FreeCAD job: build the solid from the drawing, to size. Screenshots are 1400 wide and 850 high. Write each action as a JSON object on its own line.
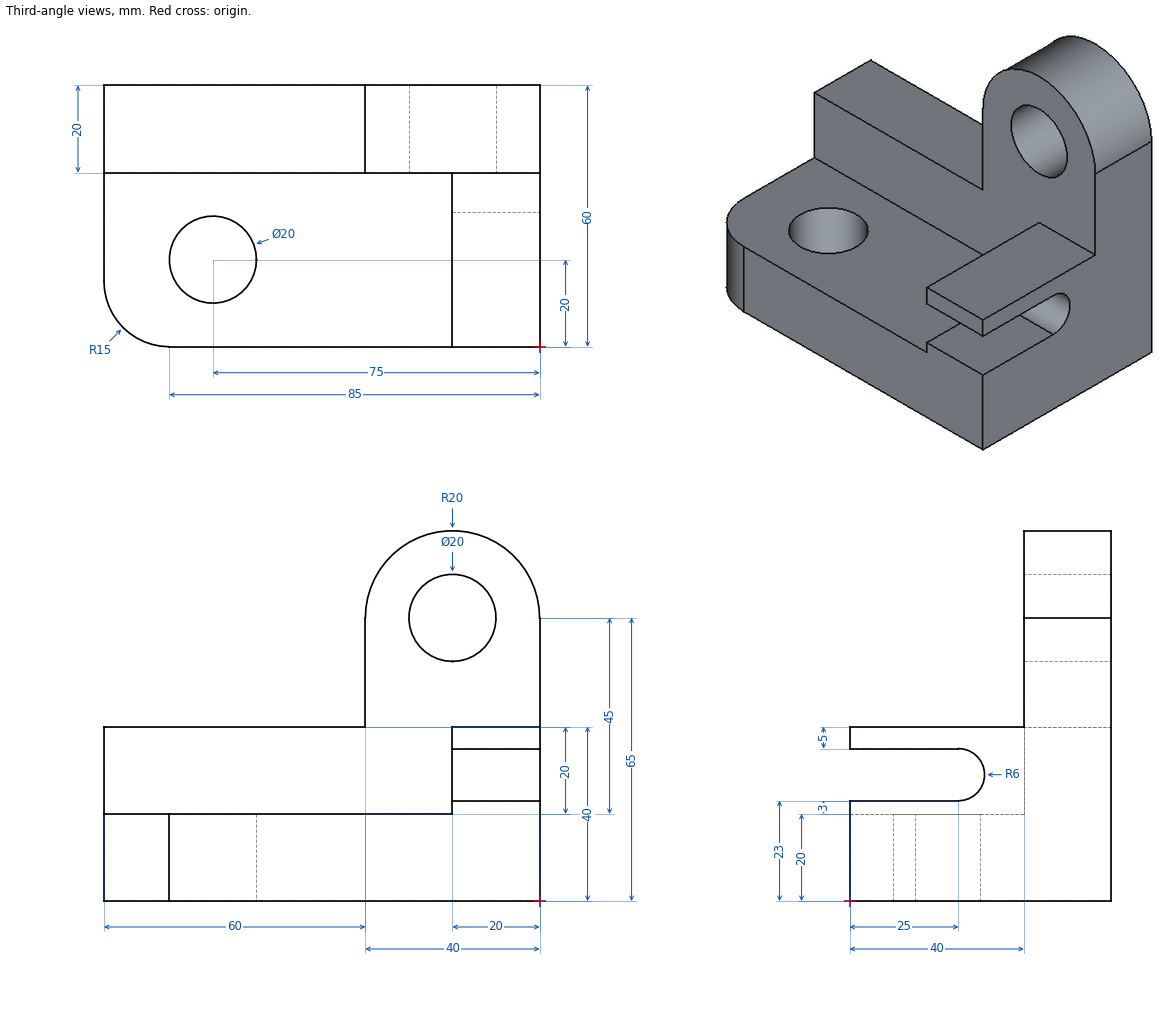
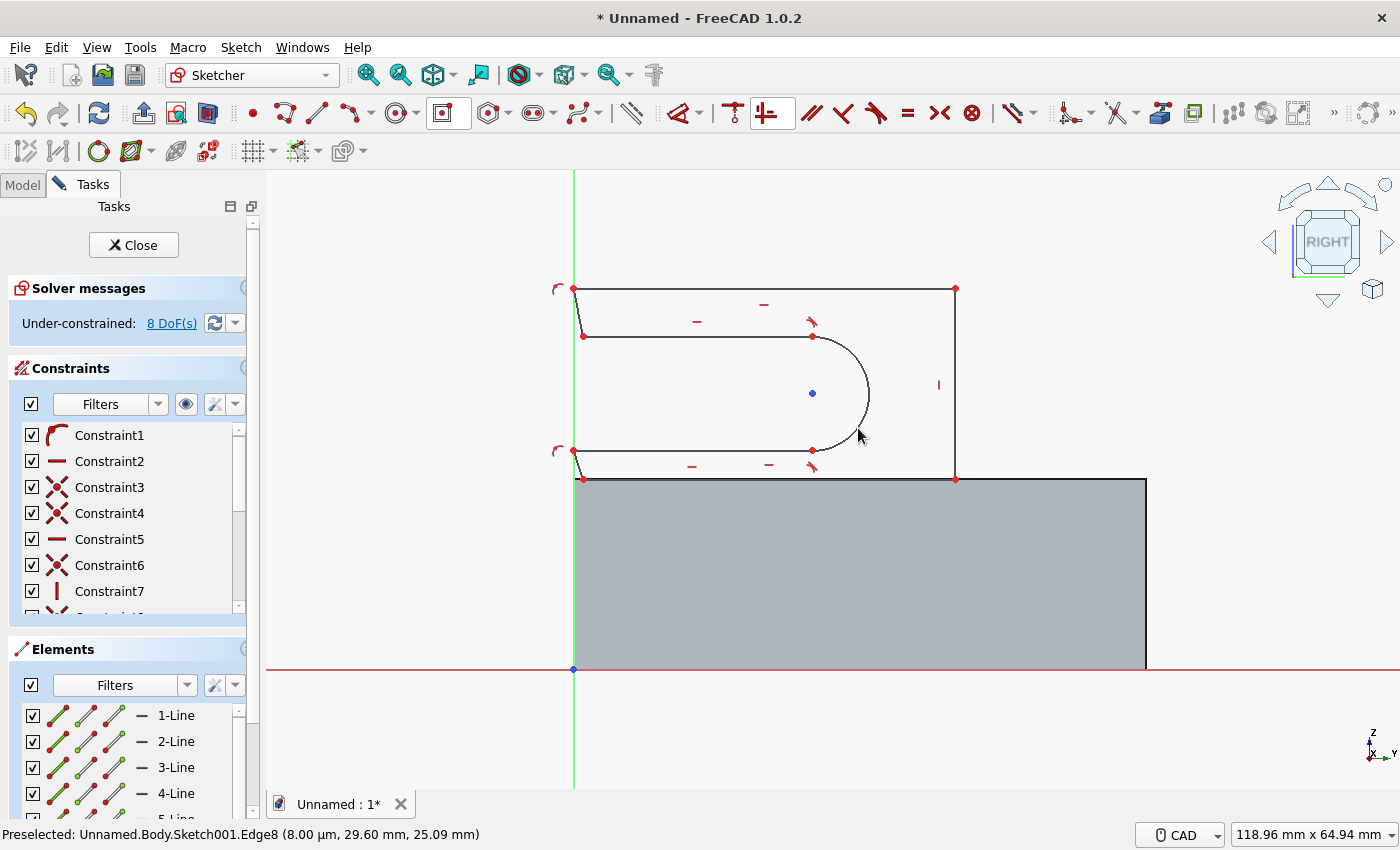
{"action": "left_click", "coordinate": [577, 463]}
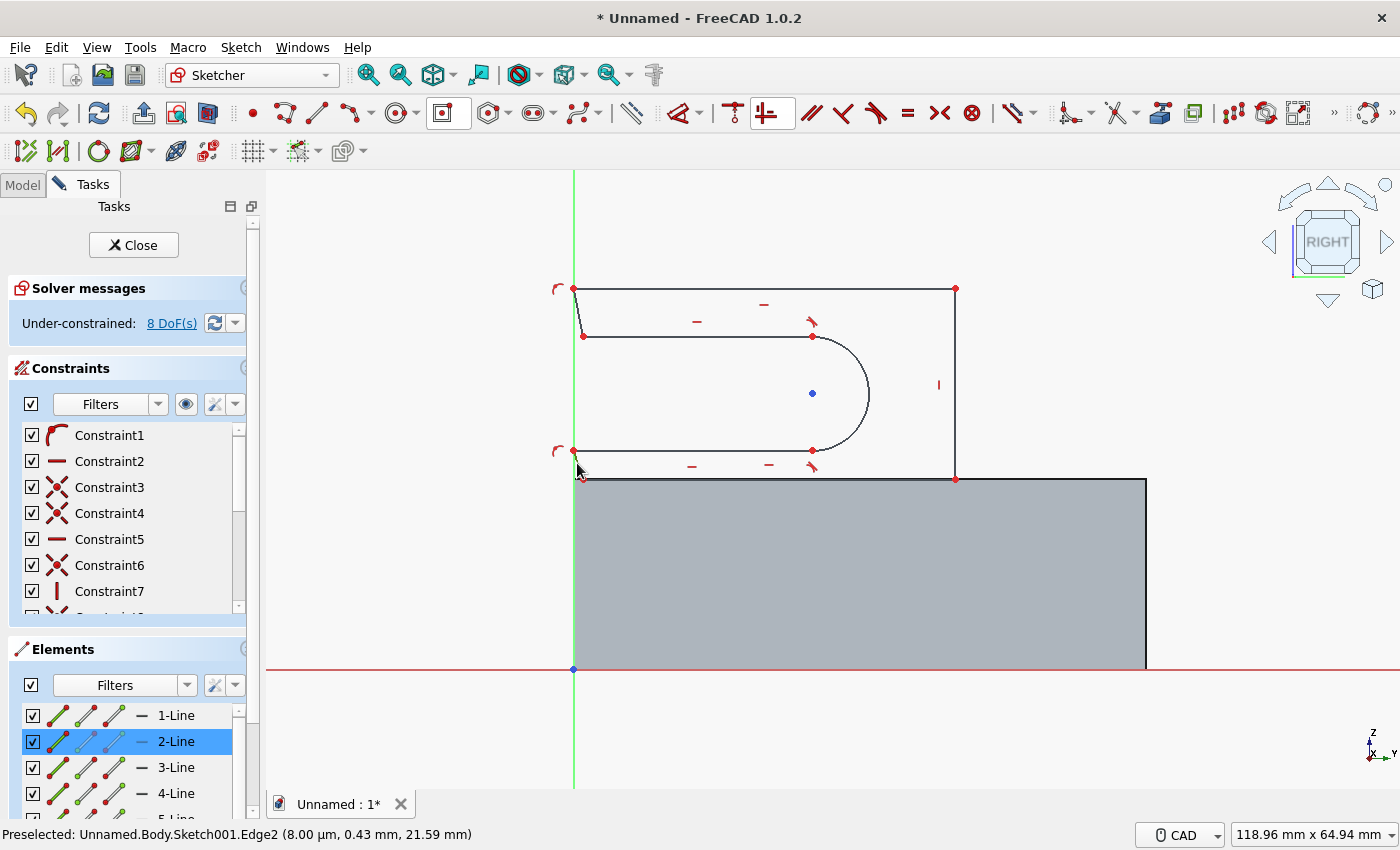
{"action": "key", "text": "v"}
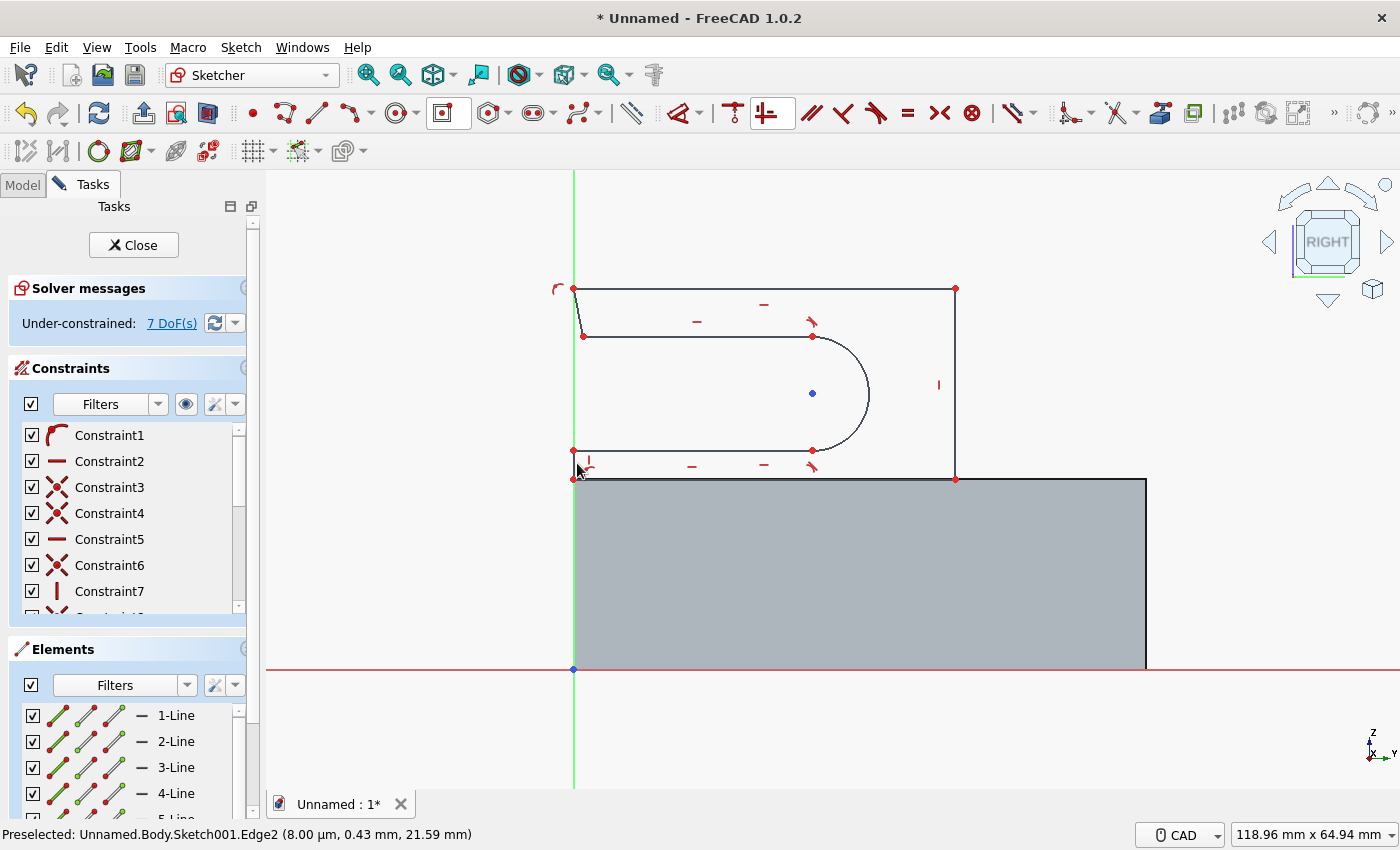
{"action": "left_click", "coordinate": [577, 303]}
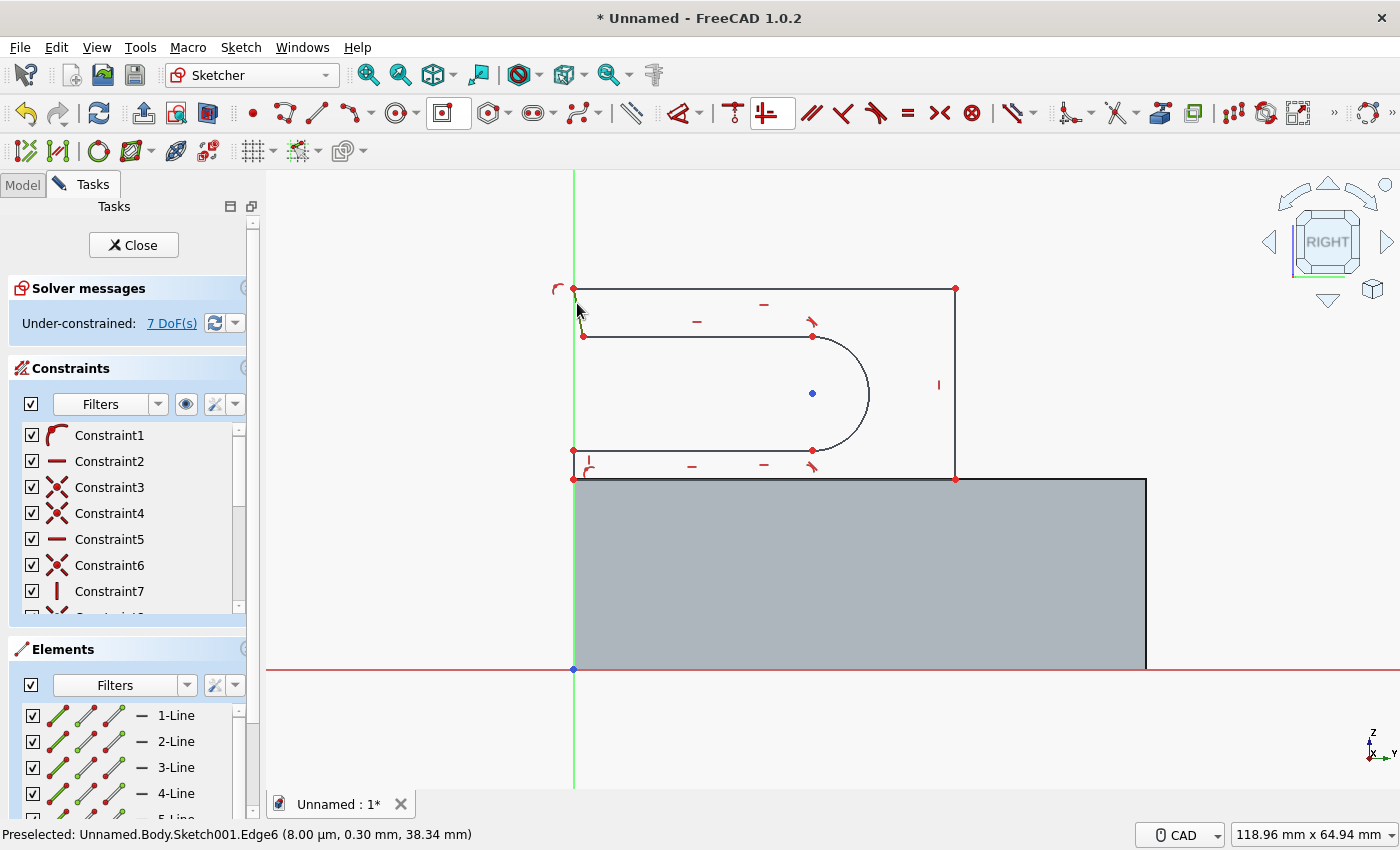
{"action": "key", "text": "v"}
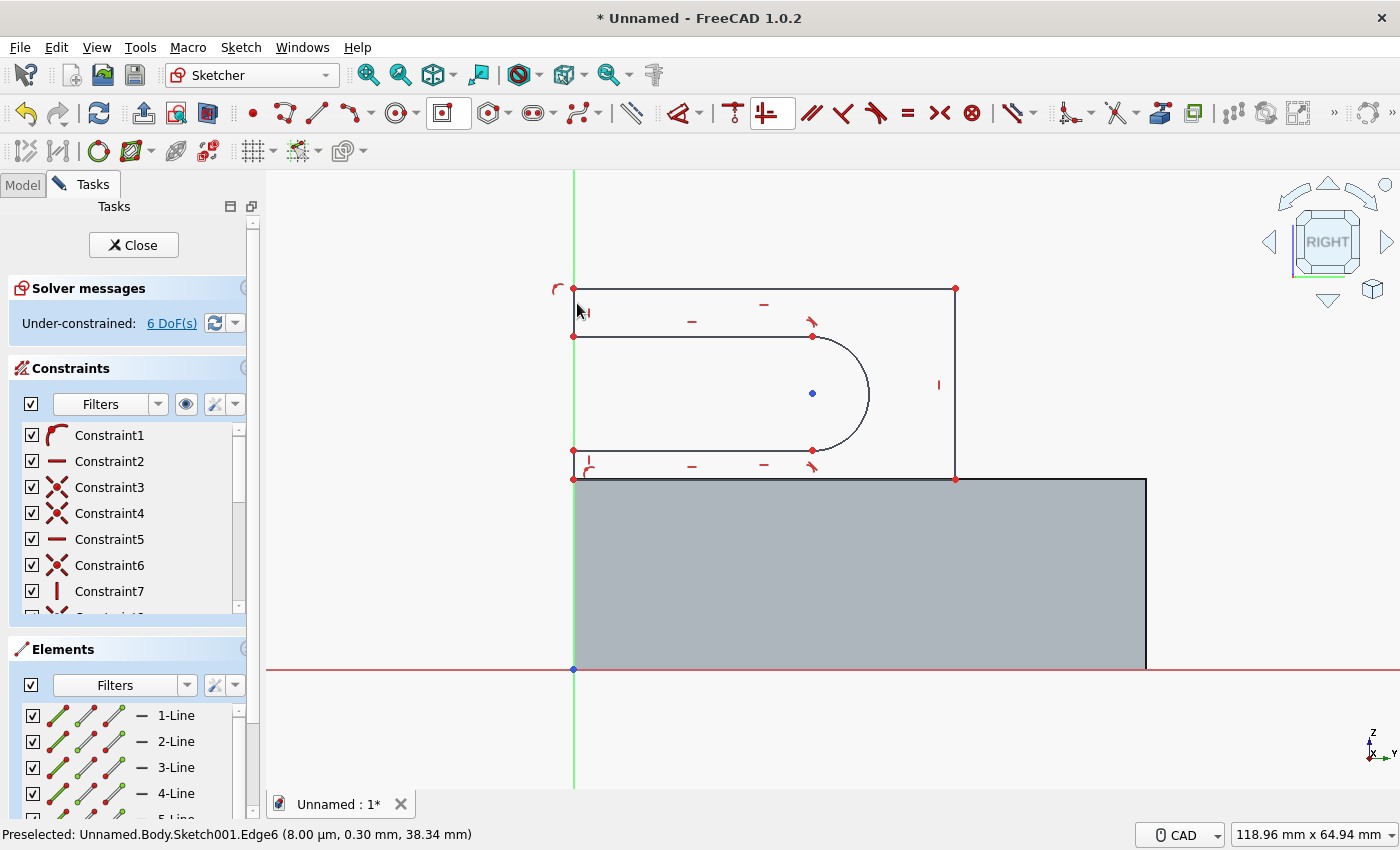
{"action": "key", "text": "d"}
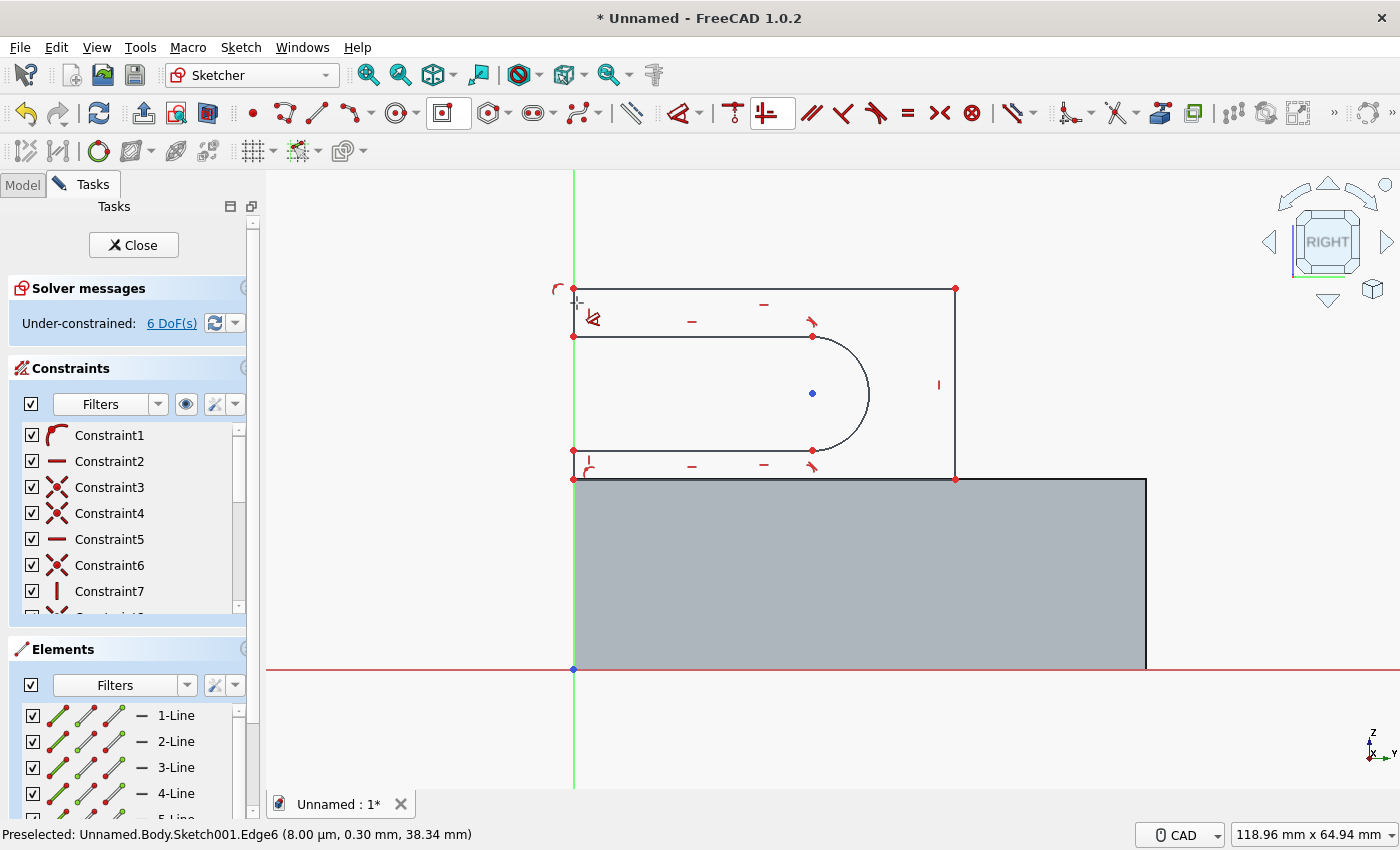
{"action": "left_click", "coordinate": [858, 428]}
{"action": "left_click", "coordinate": [884, 447]}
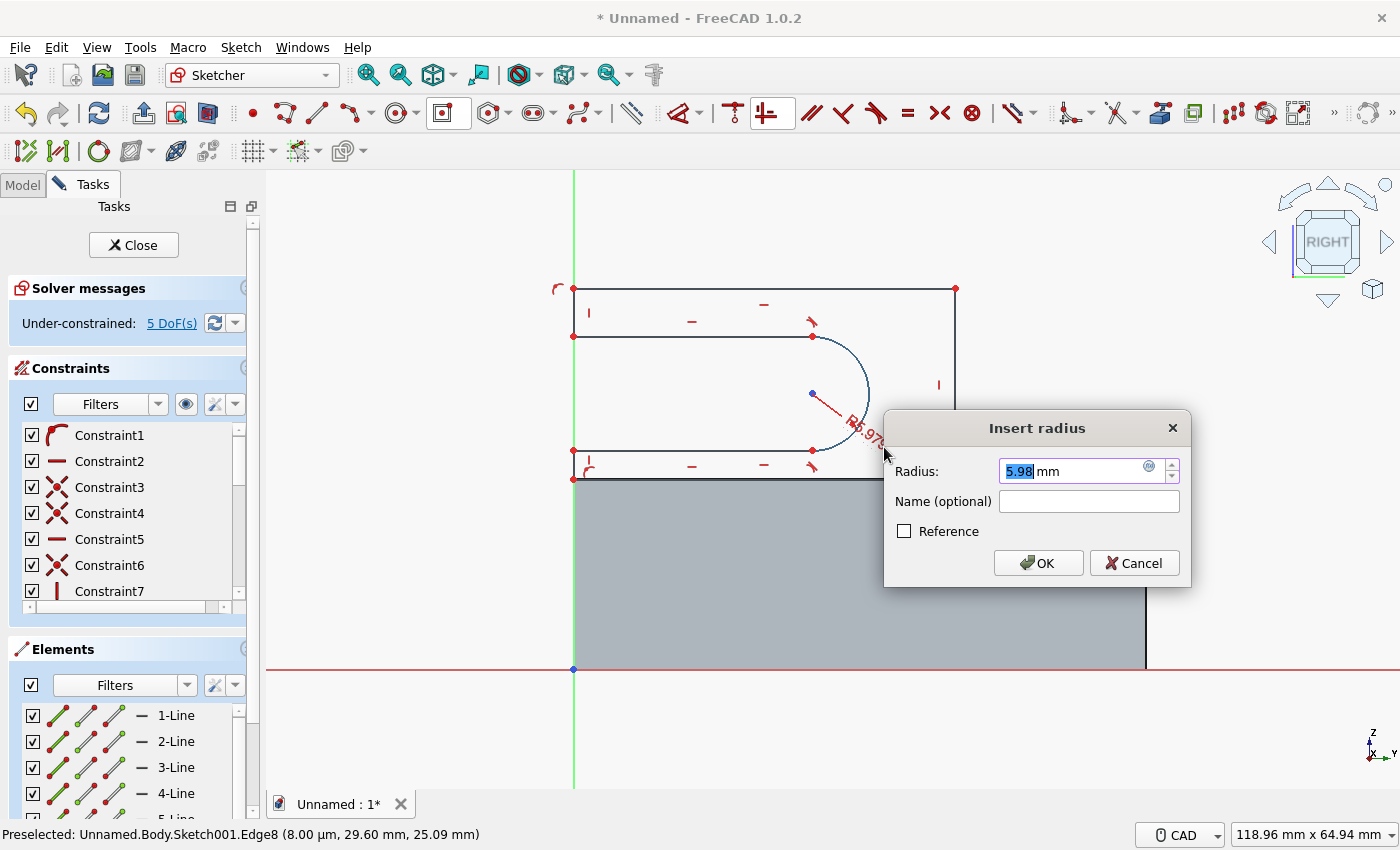
{"action": "type", "text": "6"}
{"action": "key", "text": "Return"}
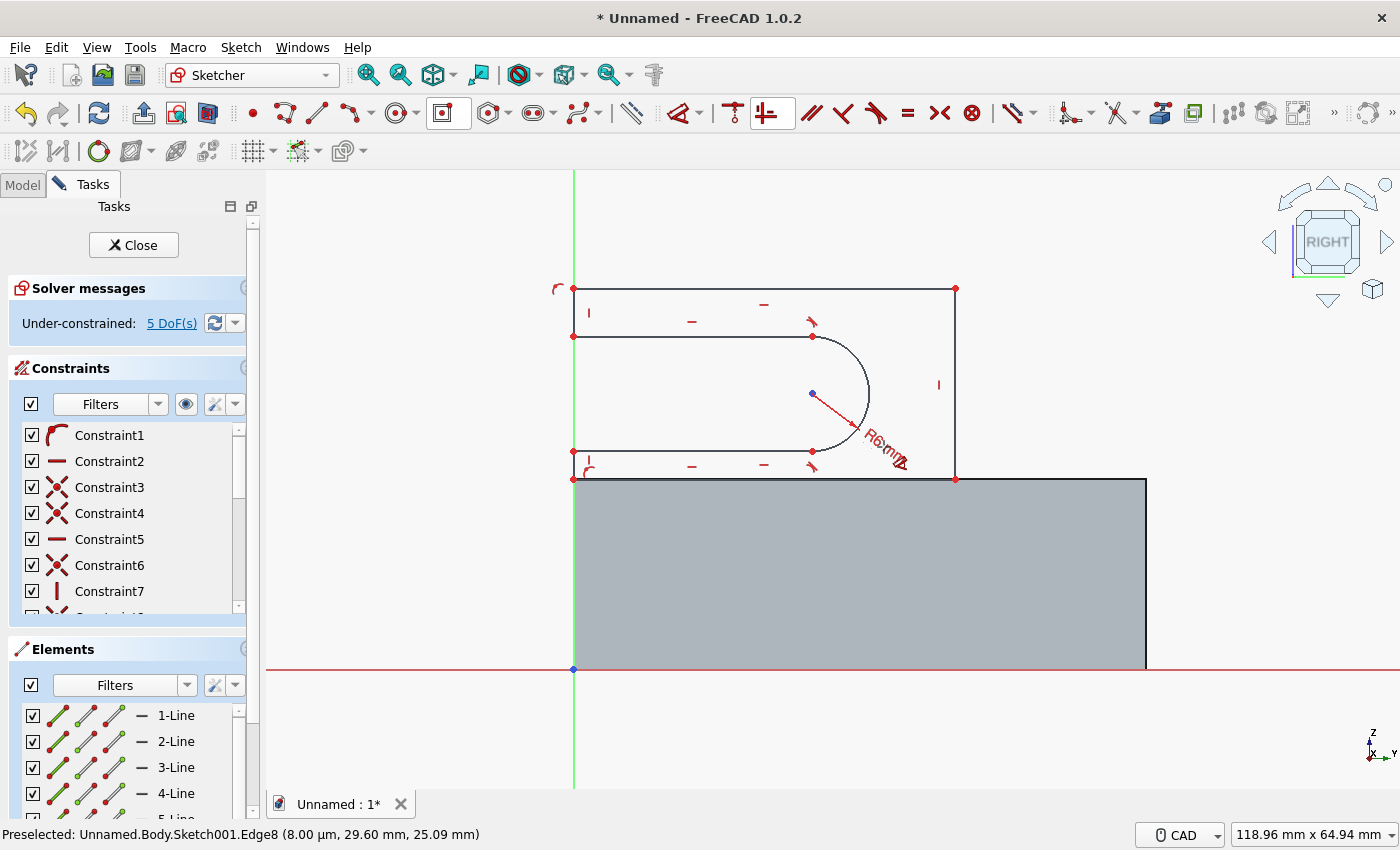
{"action": "scroll", "coordinate": [574, 463], "scroll_direction": "up", "scroll_amount": 2}